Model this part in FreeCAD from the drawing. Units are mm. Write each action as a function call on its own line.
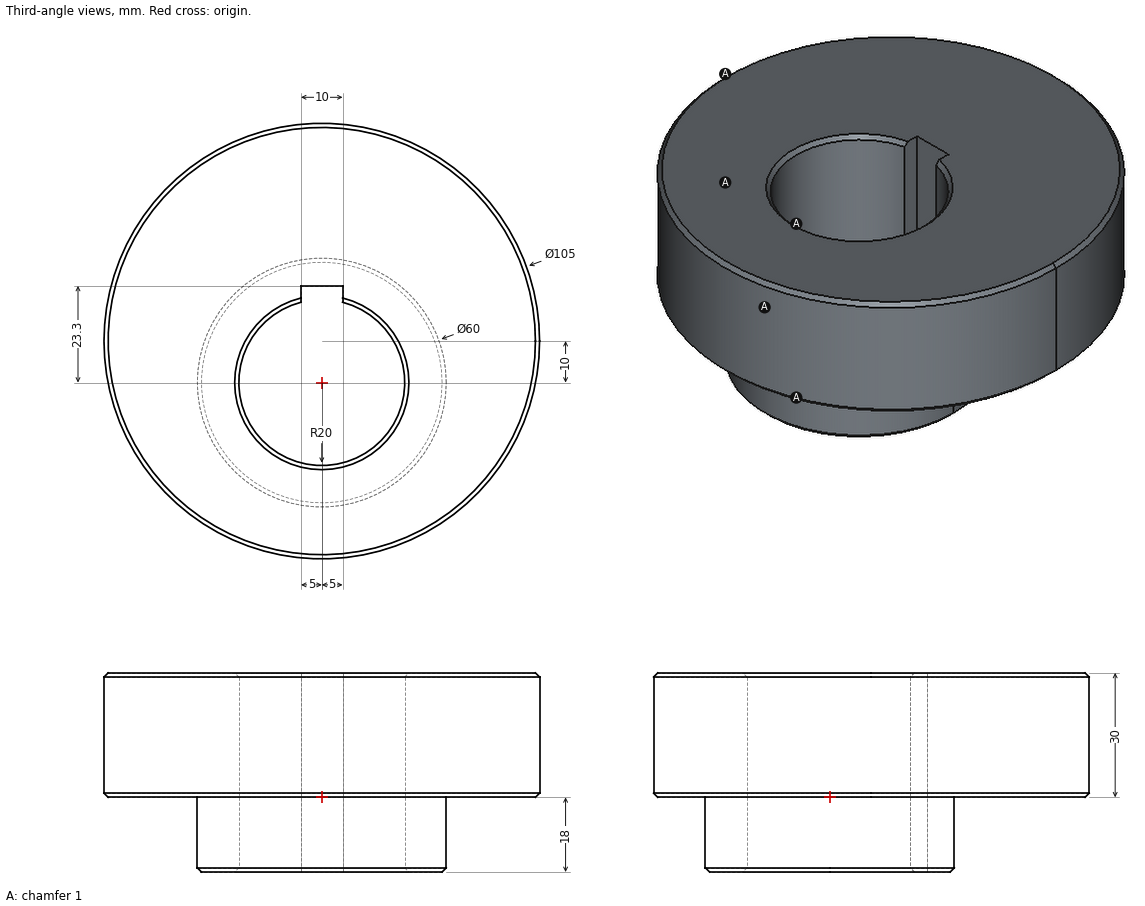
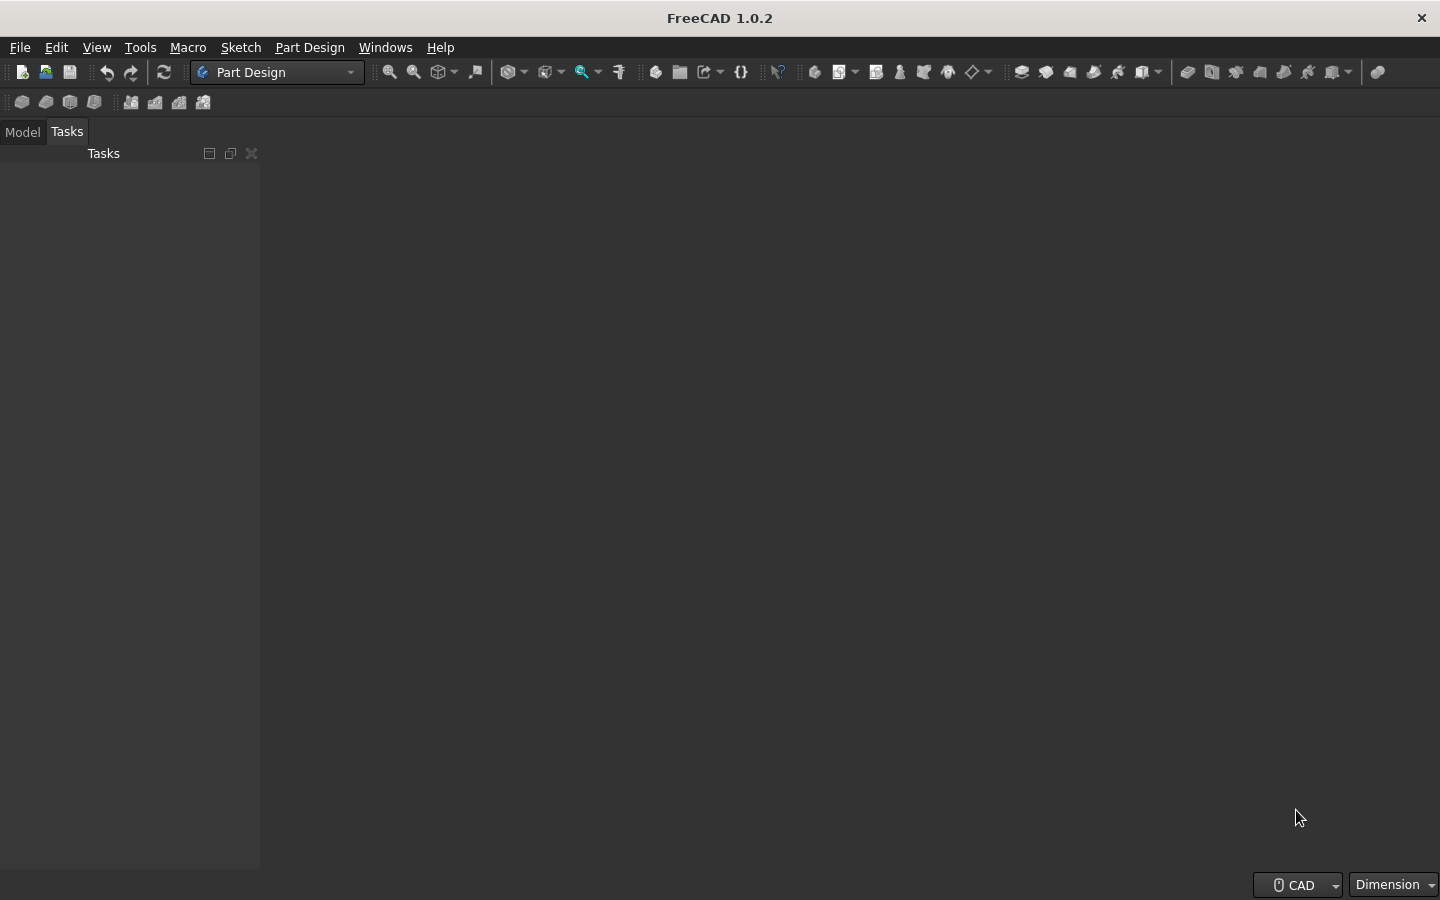
click(22, 72)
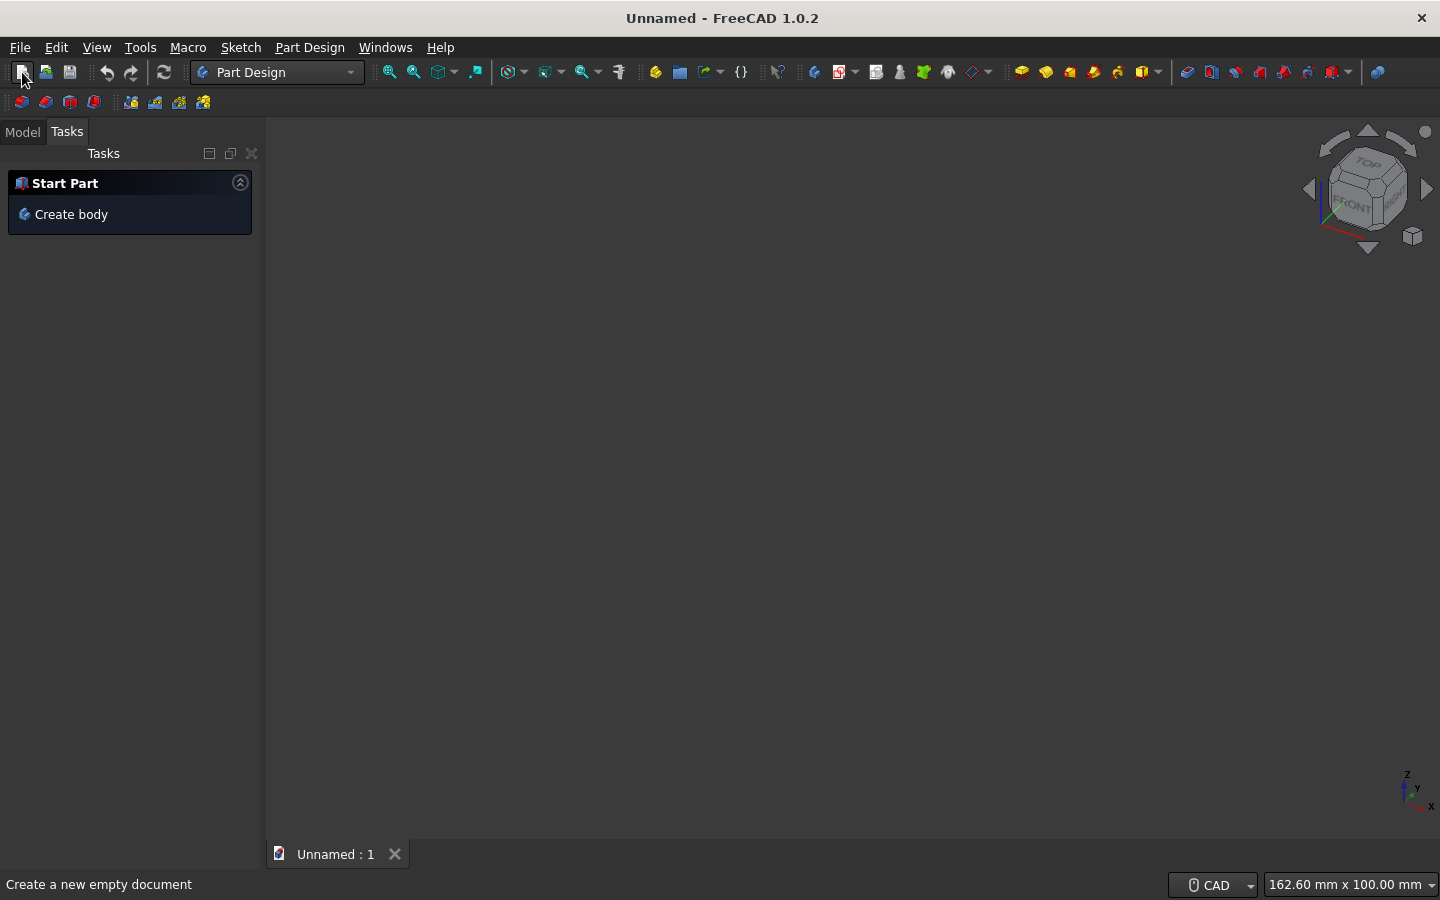
click(840, 72)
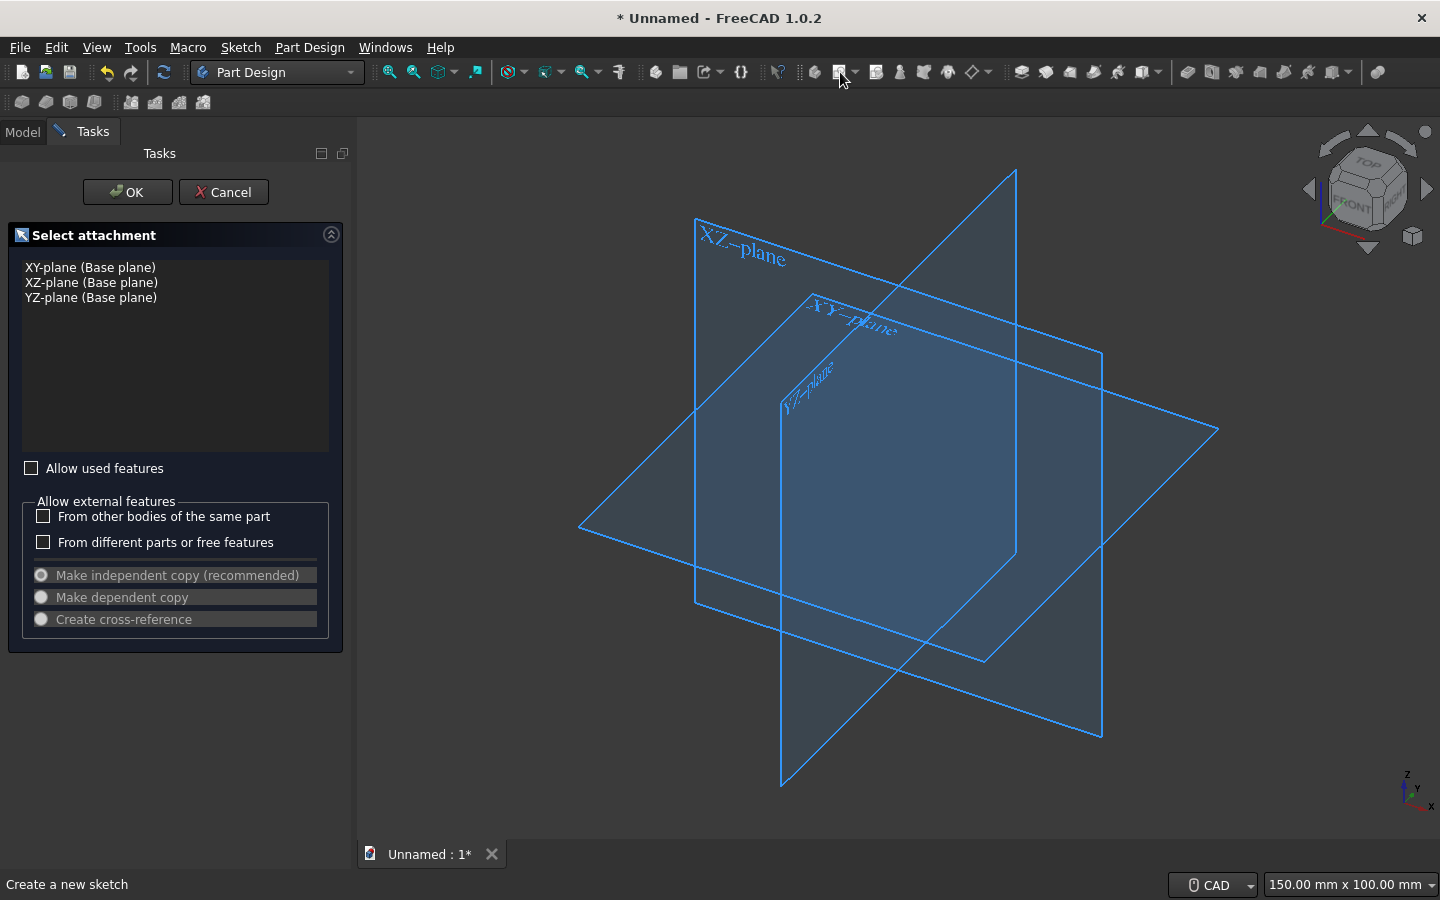
click(82, 268)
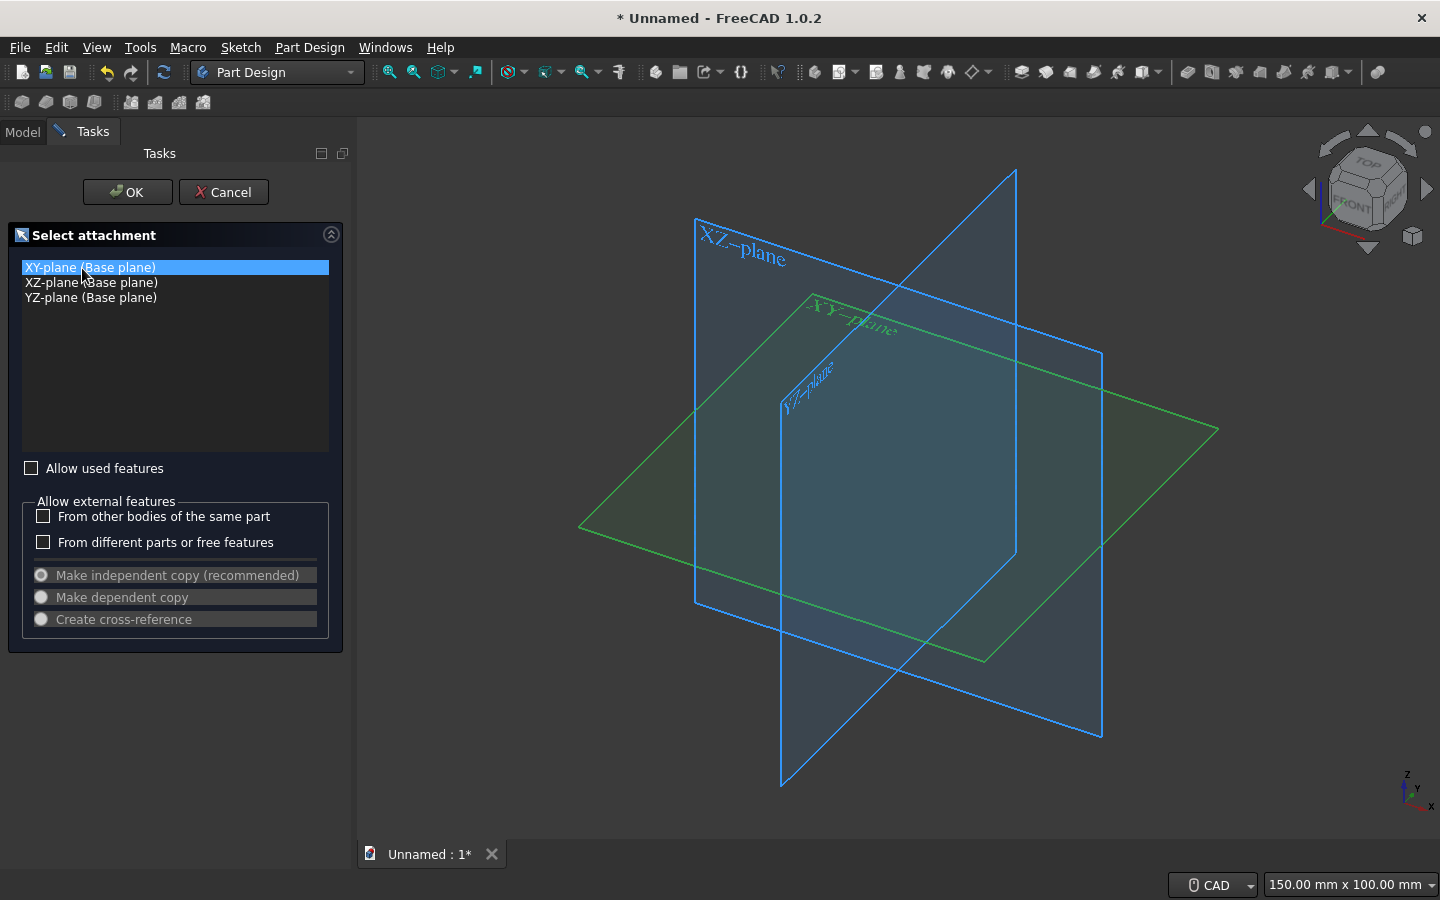
click(128, 192)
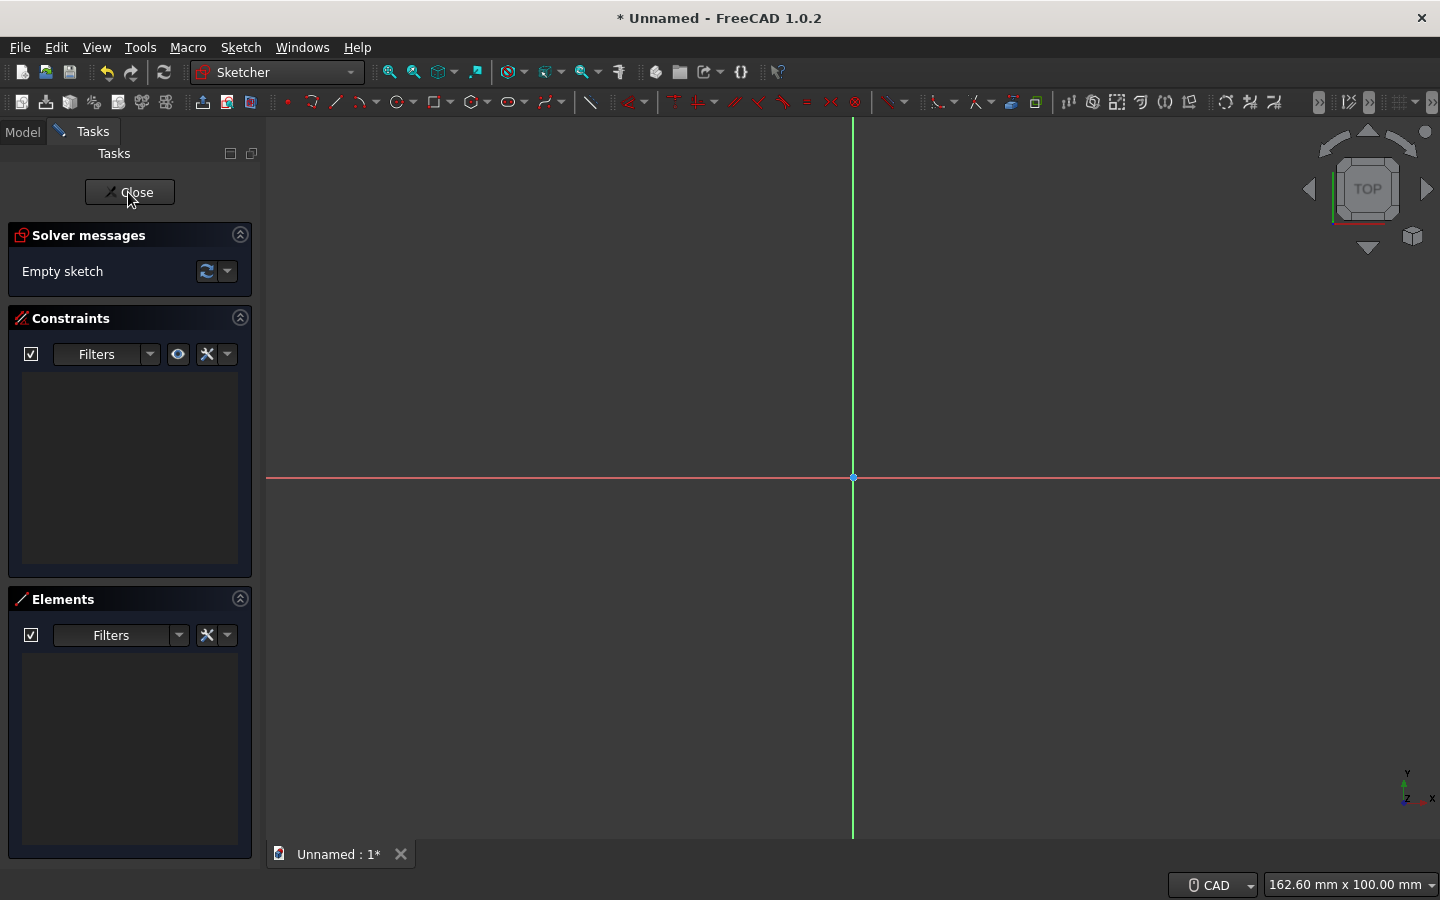
scroll(645, 625, down, 2)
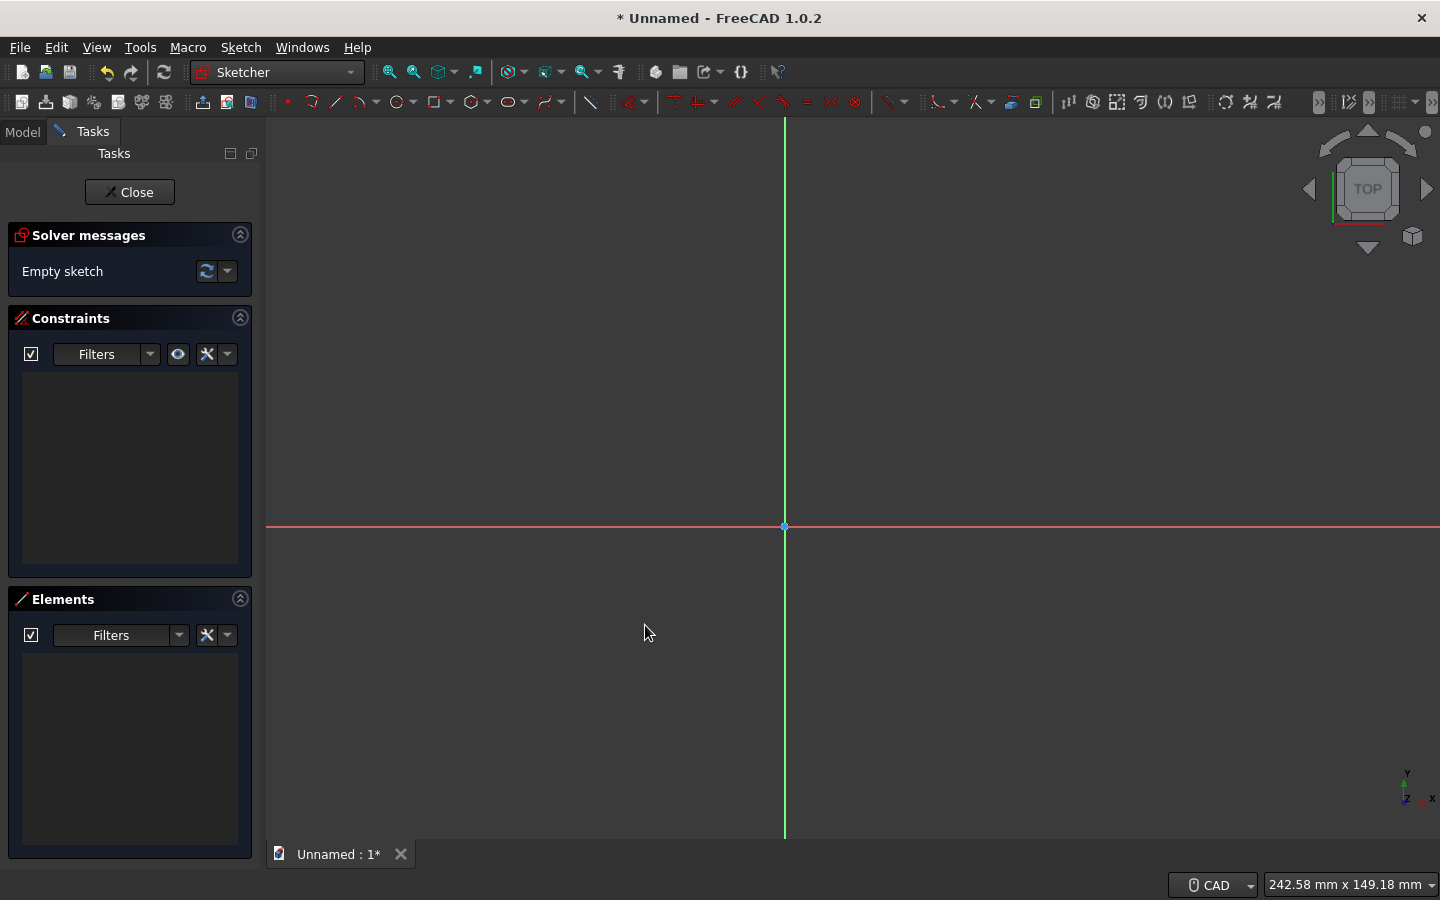
click(398, 102)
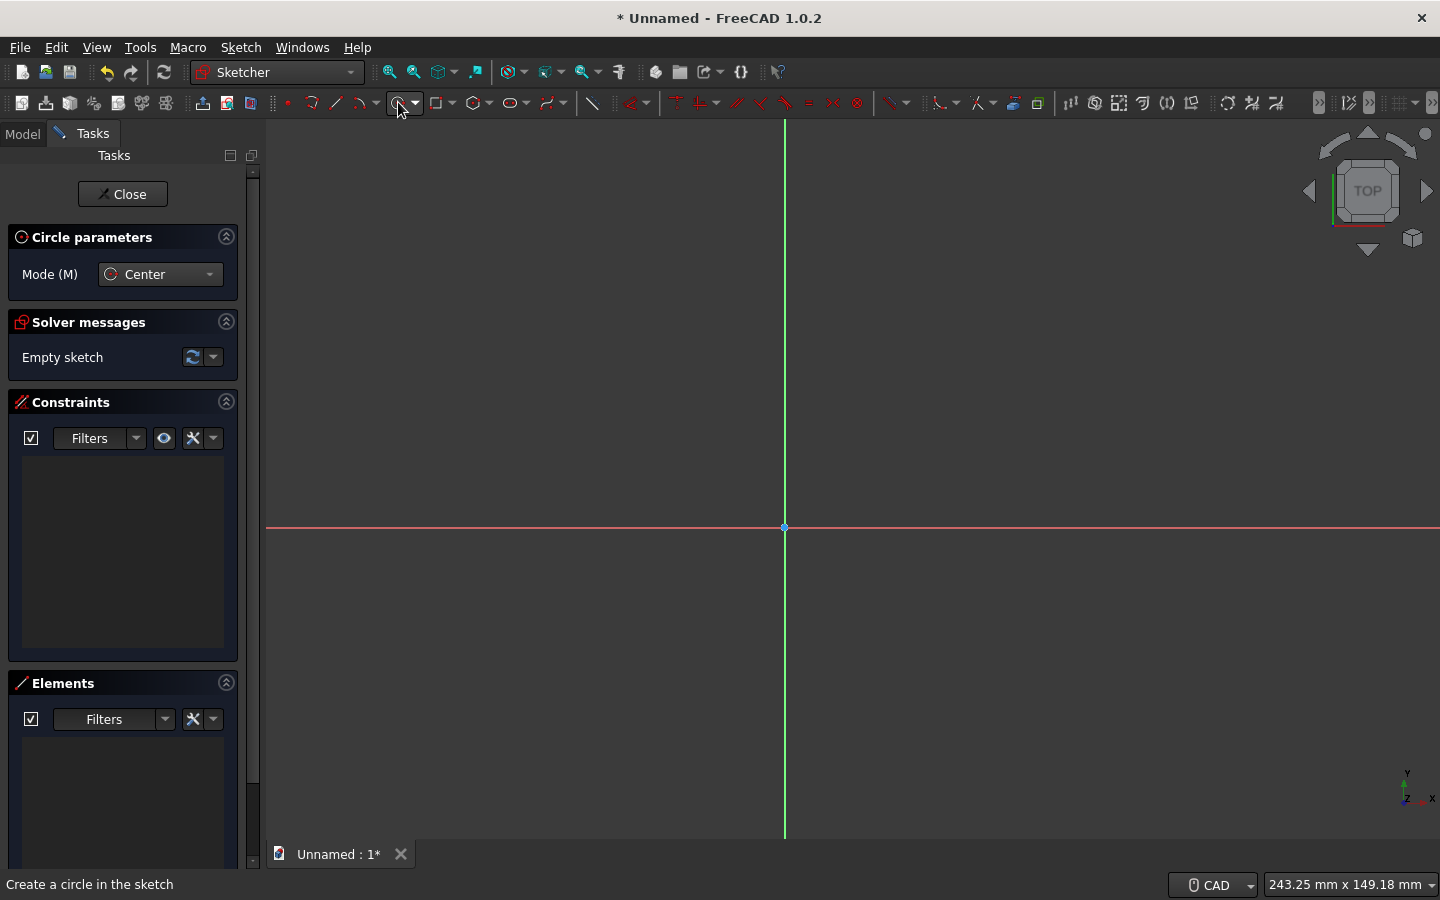
click(785, 479)
move(964, 300)